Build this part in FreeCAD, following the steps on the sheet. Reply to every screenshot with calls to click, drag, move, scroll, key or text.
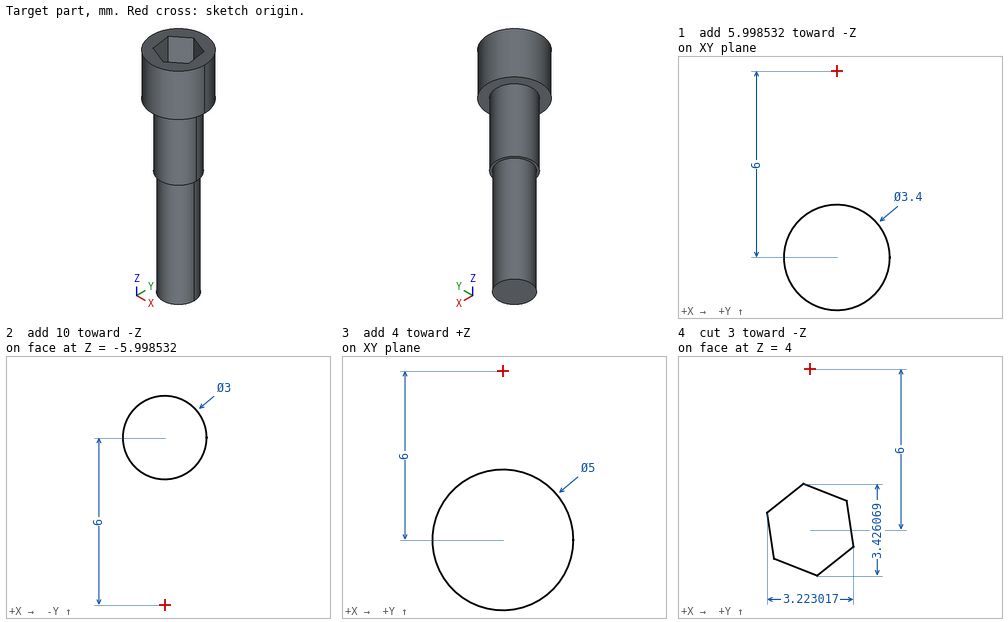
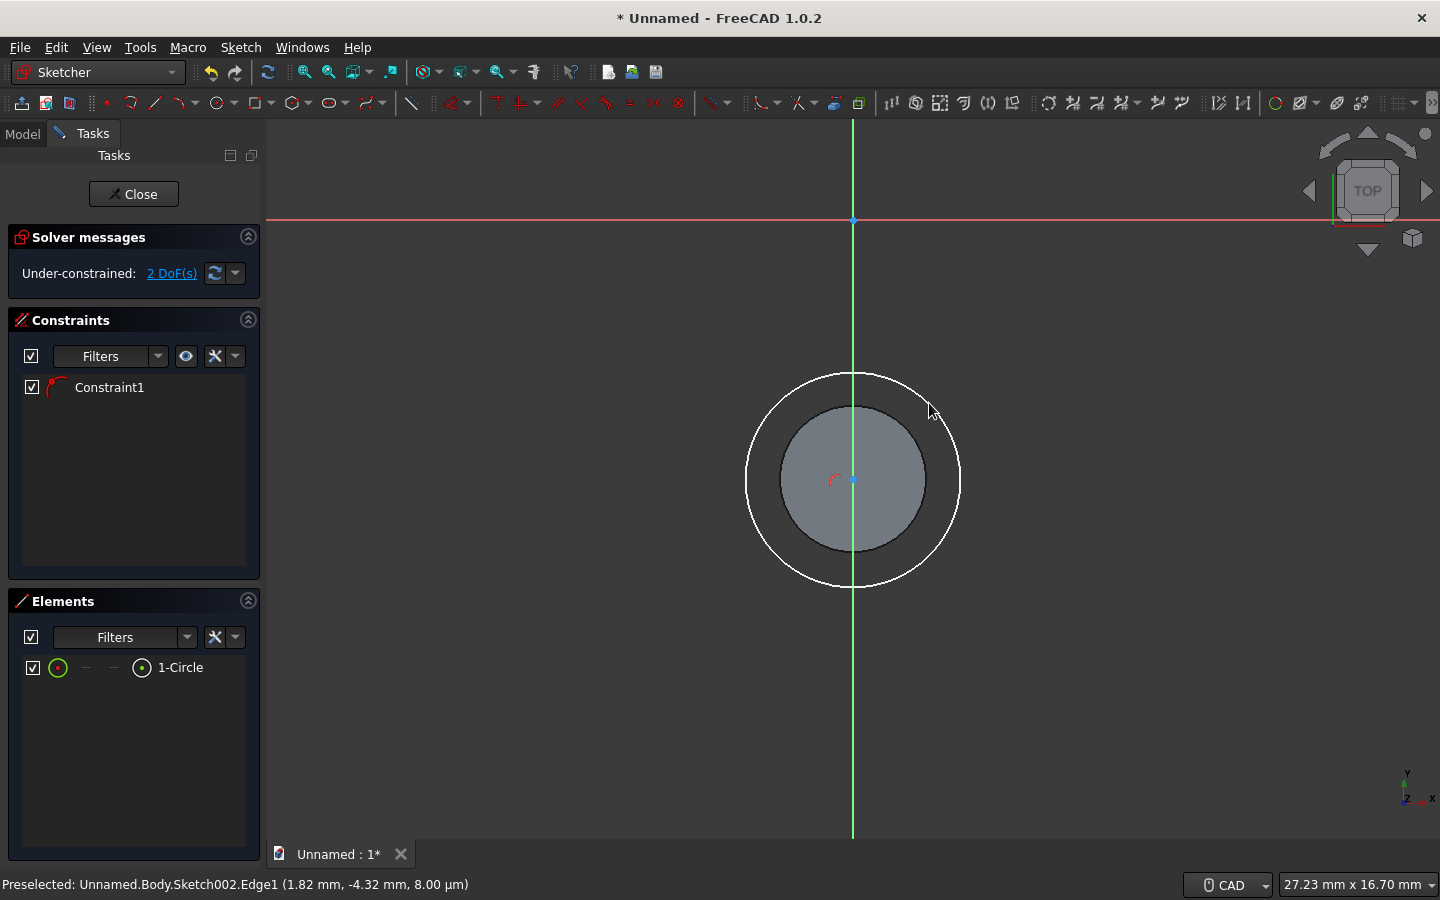
key(d)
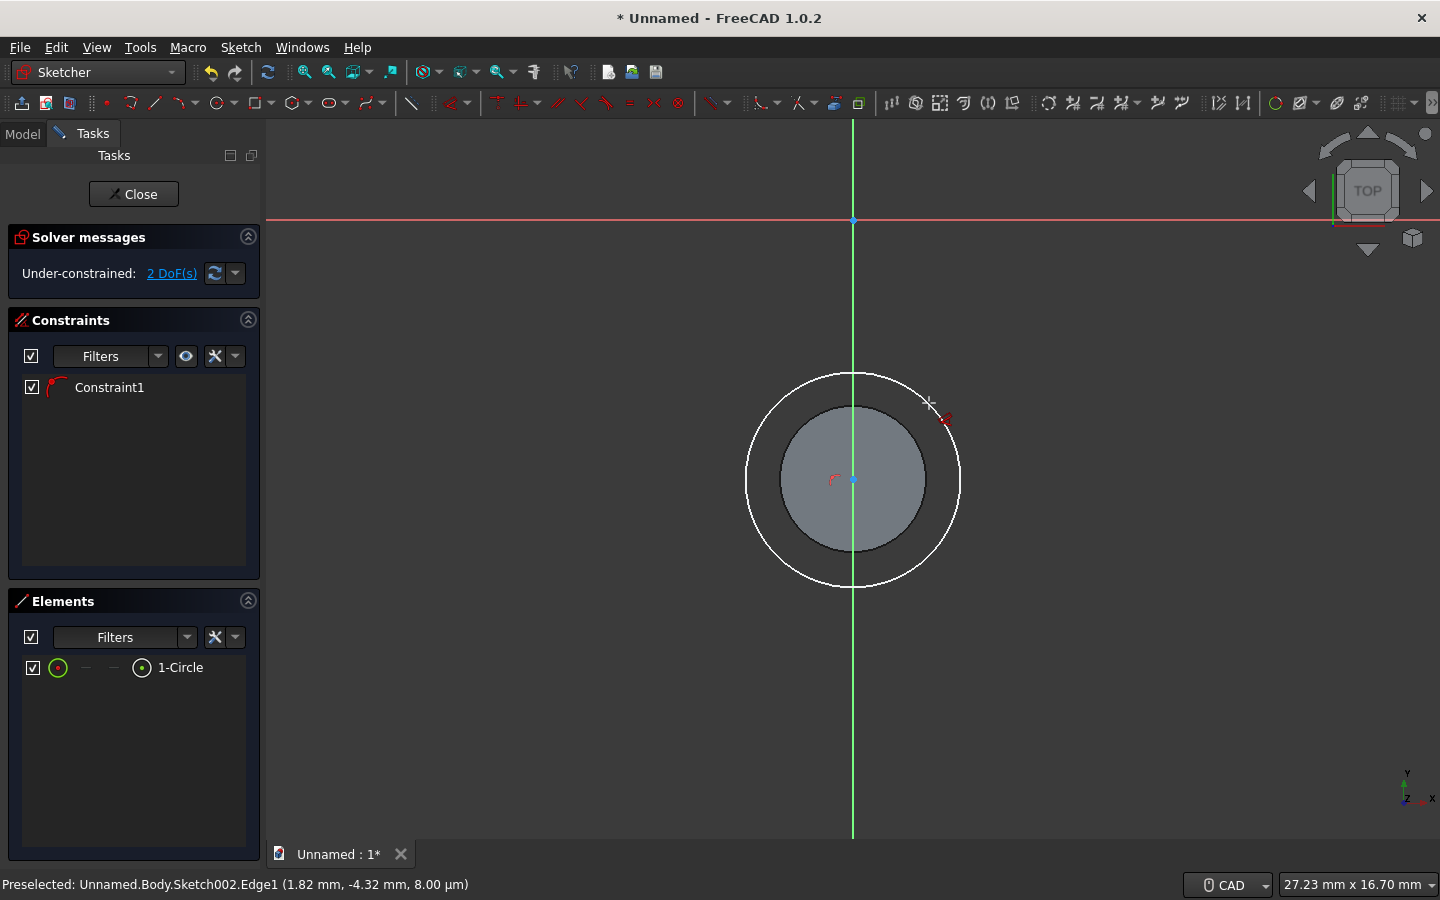
click(929, 404)
click(952, 381)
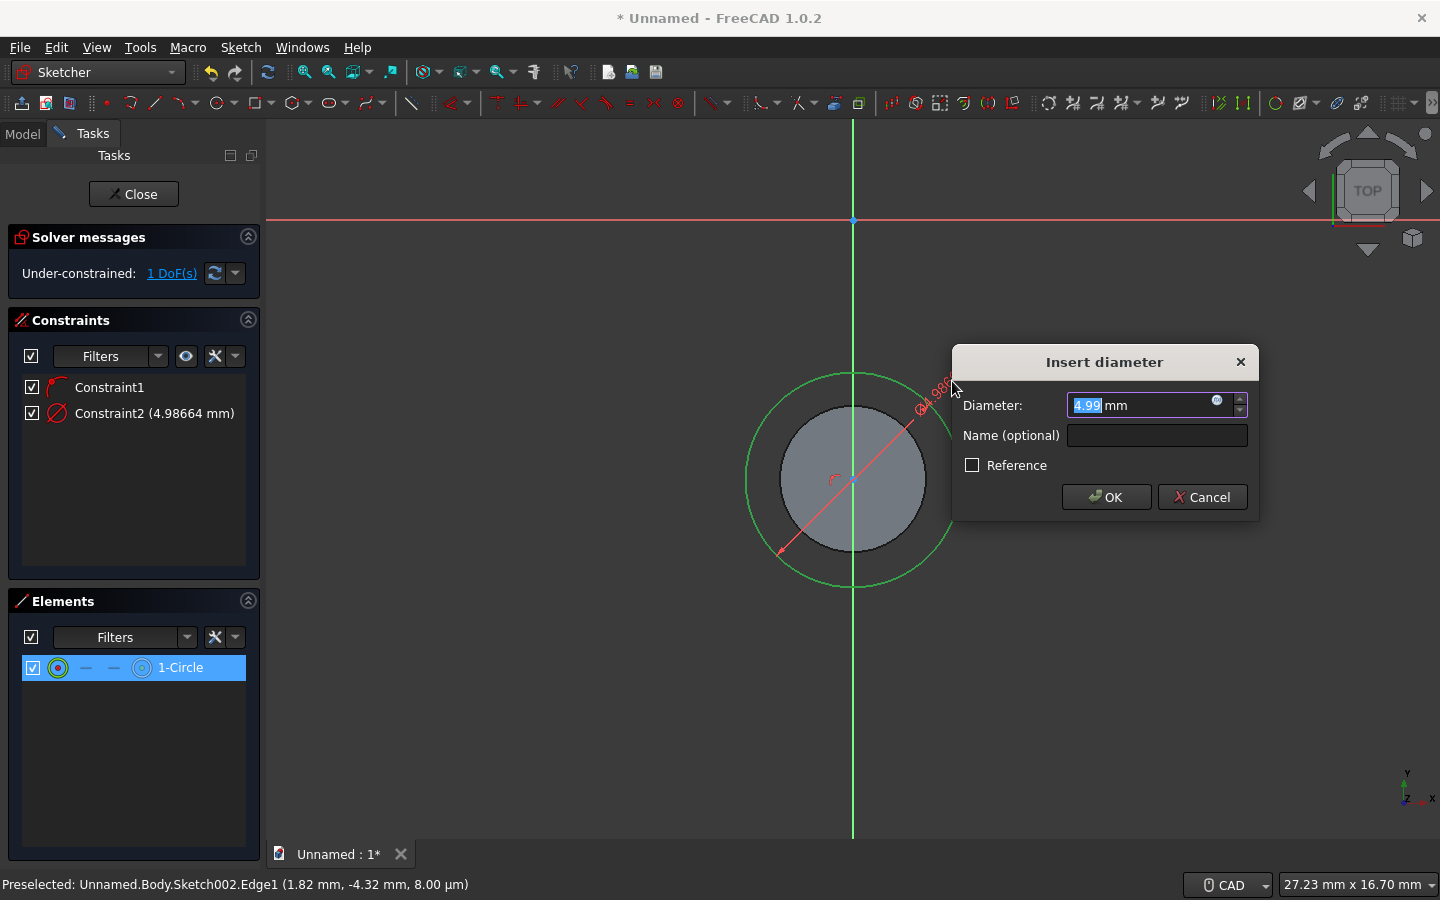
text(5)
key(Return)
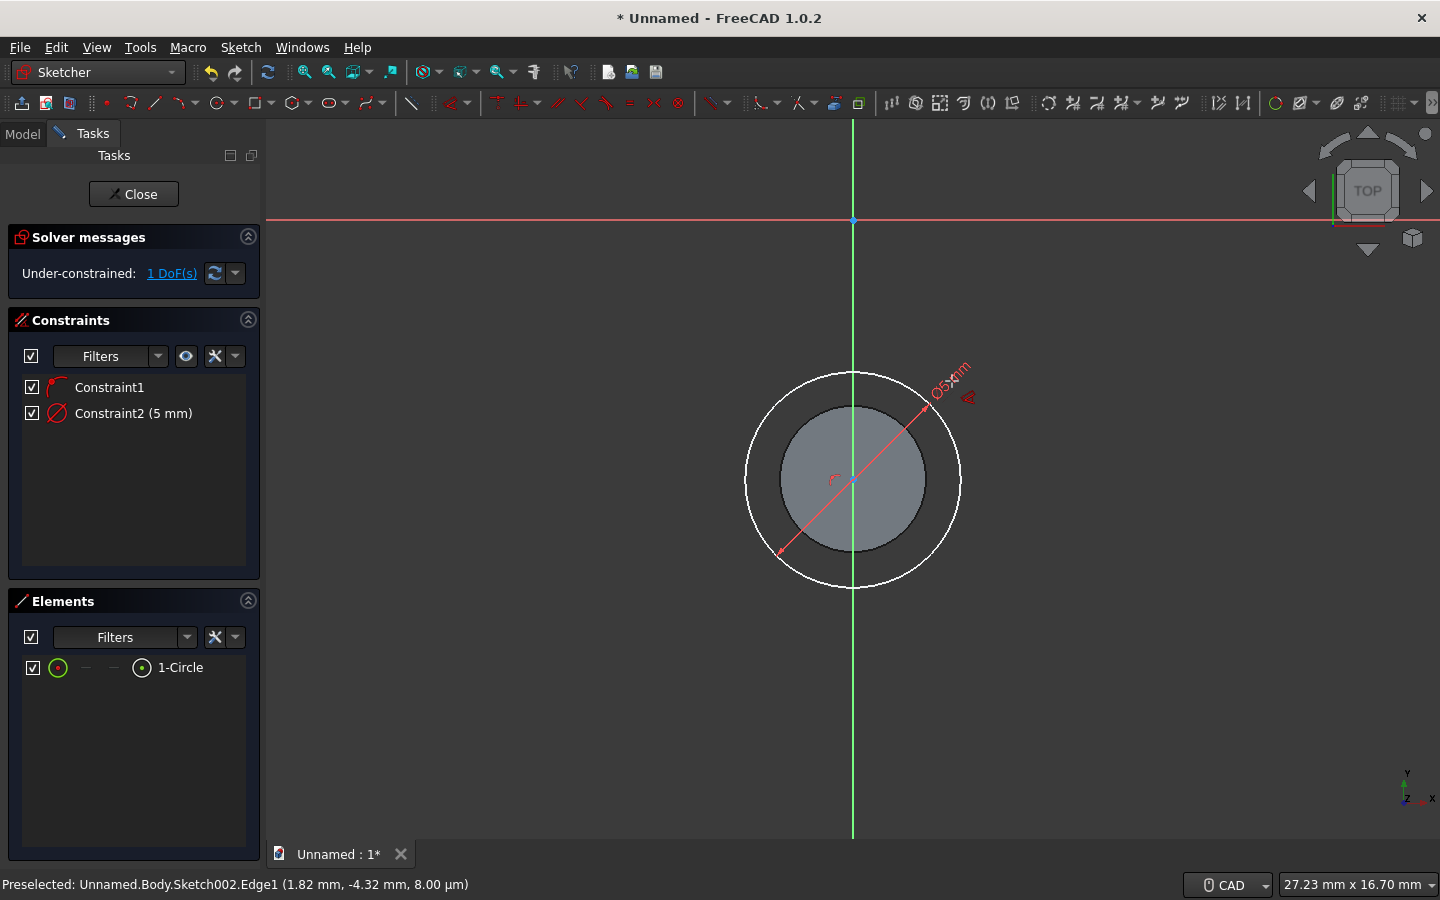
scroll(853, 480, up, 4)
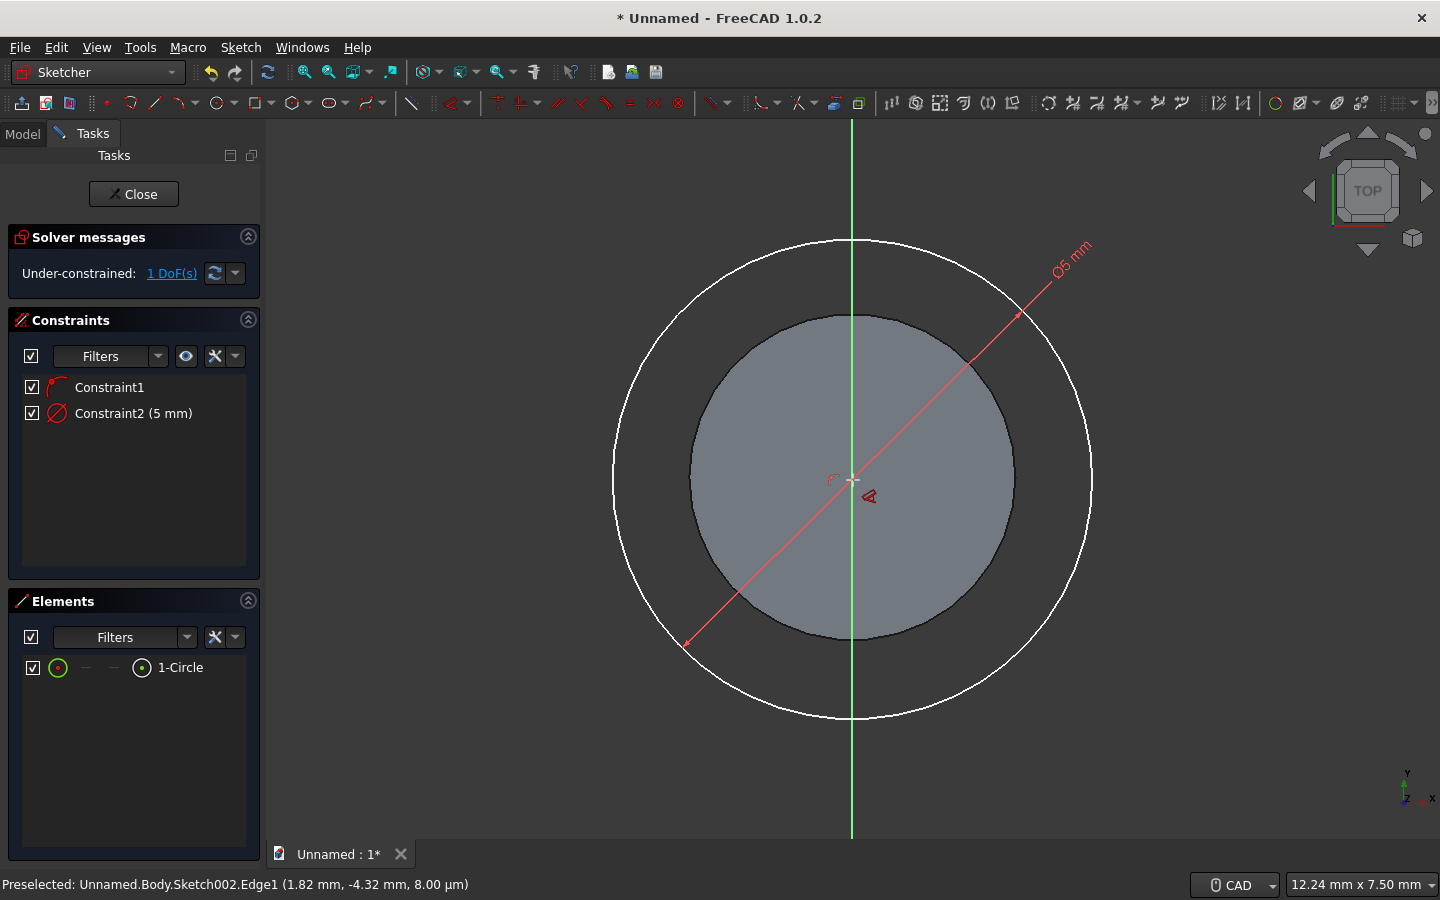
scroll(852, 479, up, 4)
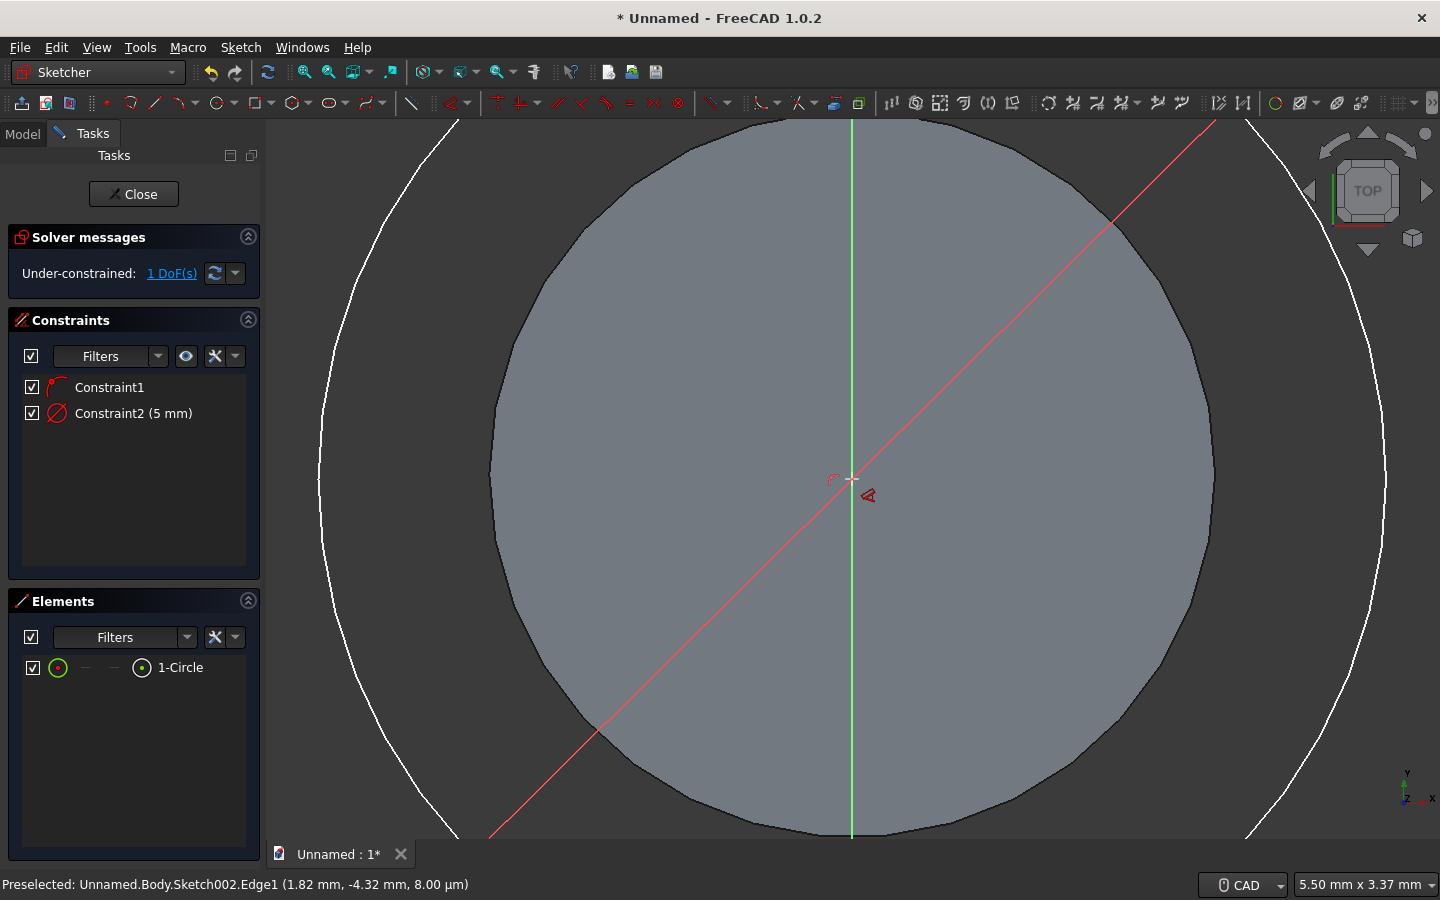
click(852, 479)
click(886, 313)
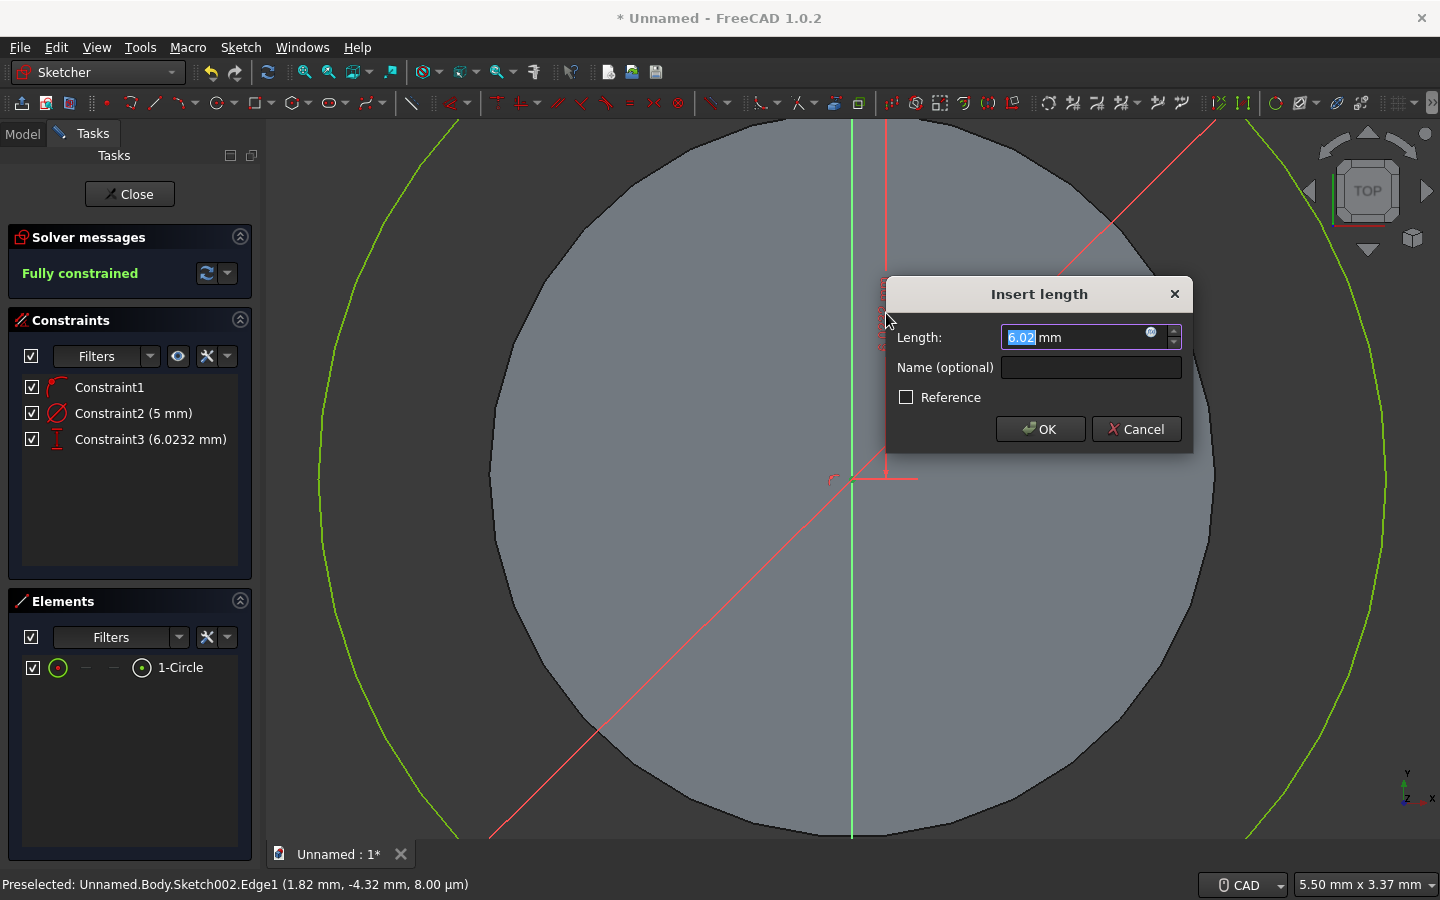
text(6)
key(Return)
key(Escape)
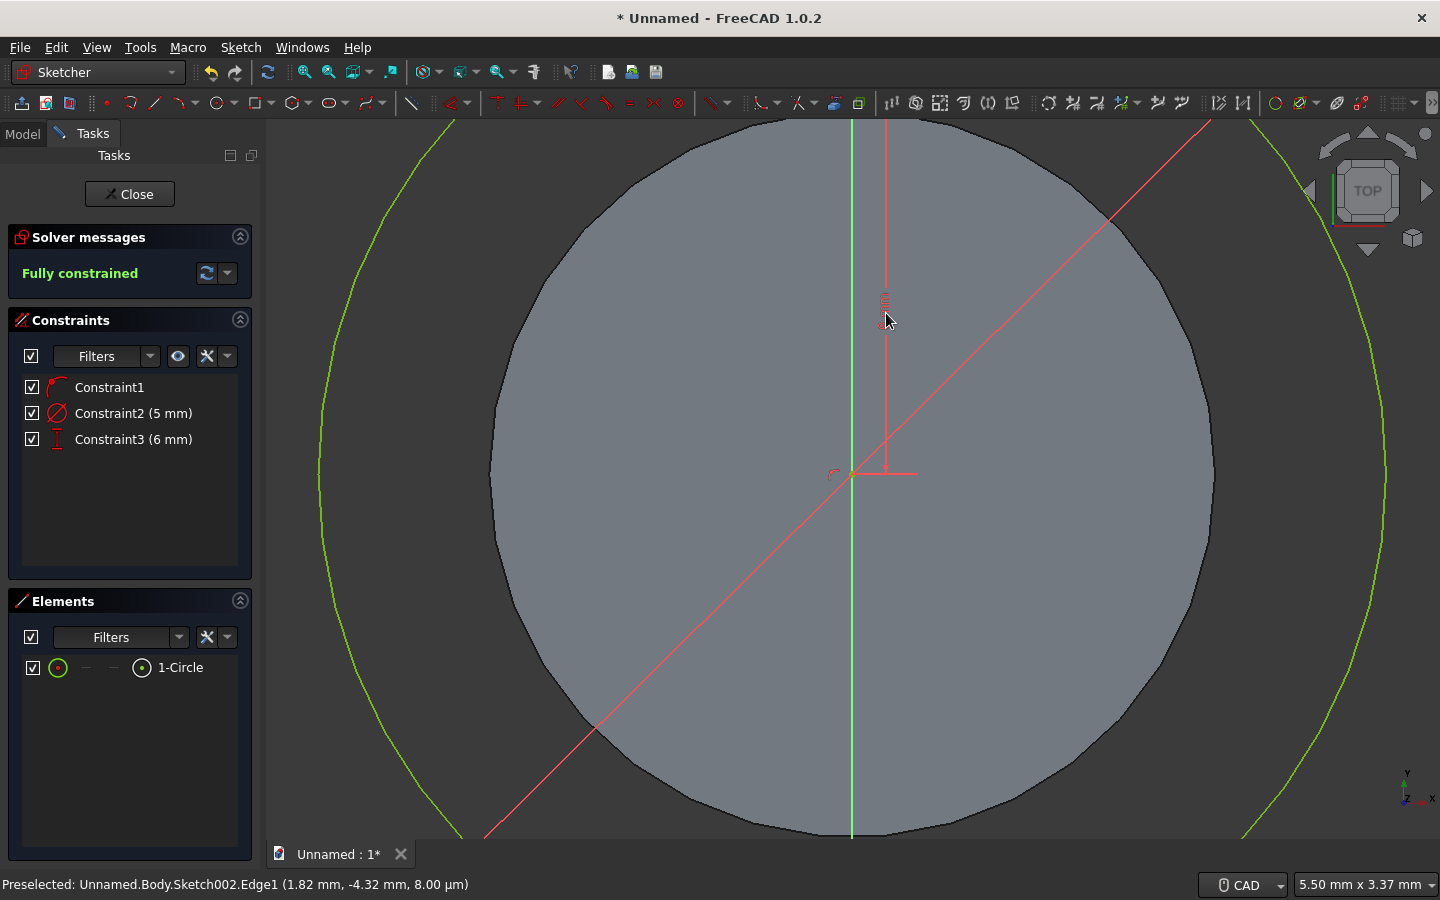
click(130, 194)